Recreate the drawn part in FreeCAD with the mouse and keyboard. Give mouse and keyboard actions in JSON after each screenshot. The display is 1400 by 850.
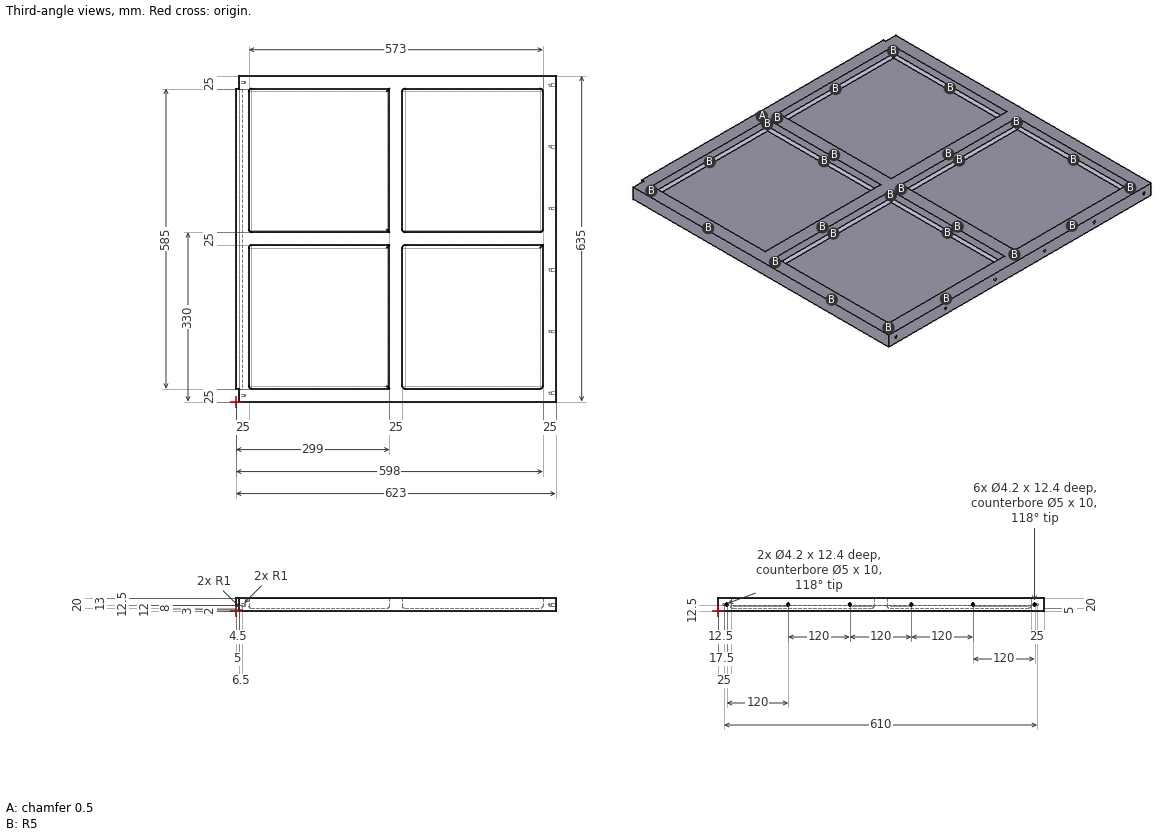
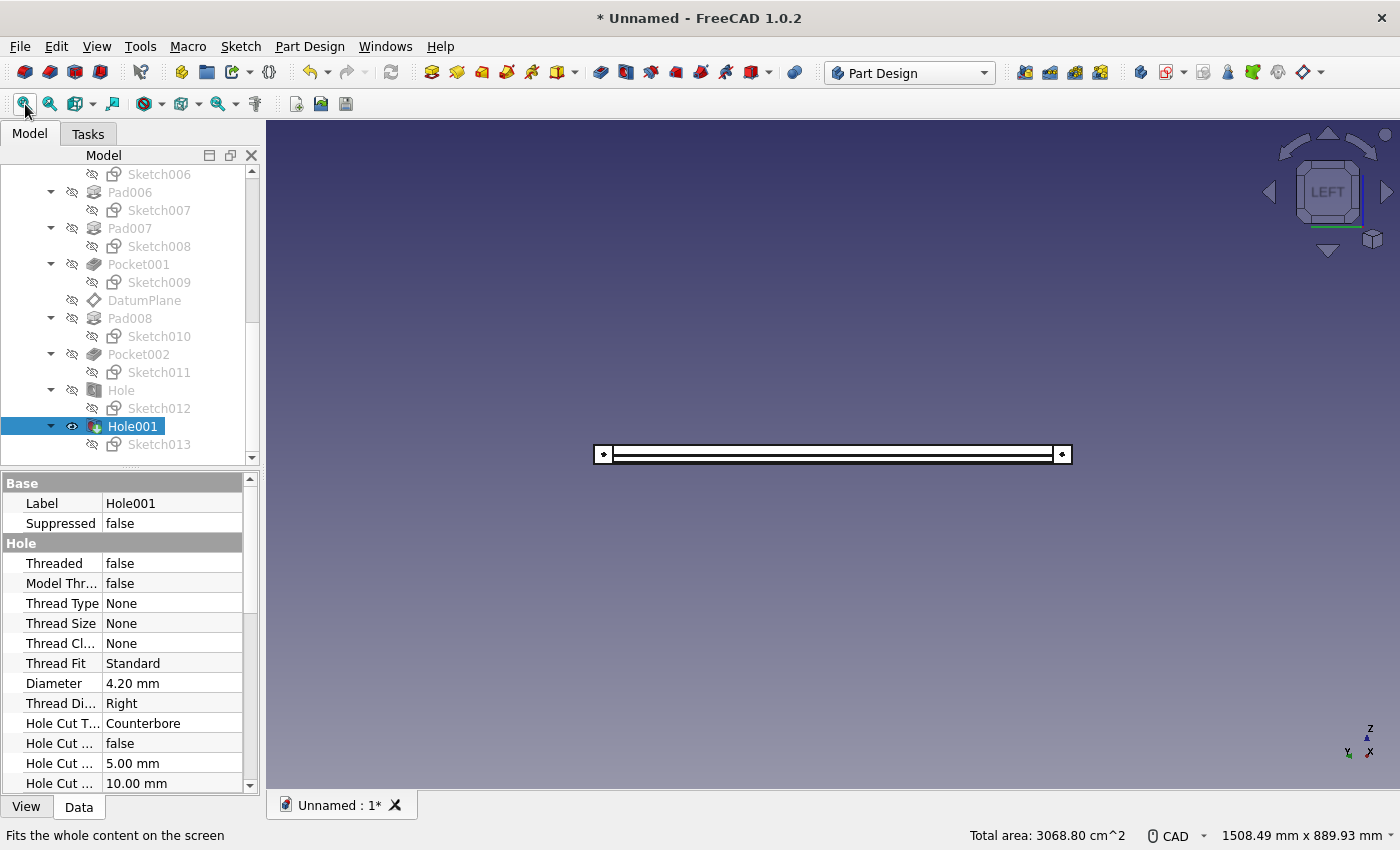
{"action": "scroll", "coordinate": [1053, 452], "scroll_direction": "up", "scroll_amount": 5}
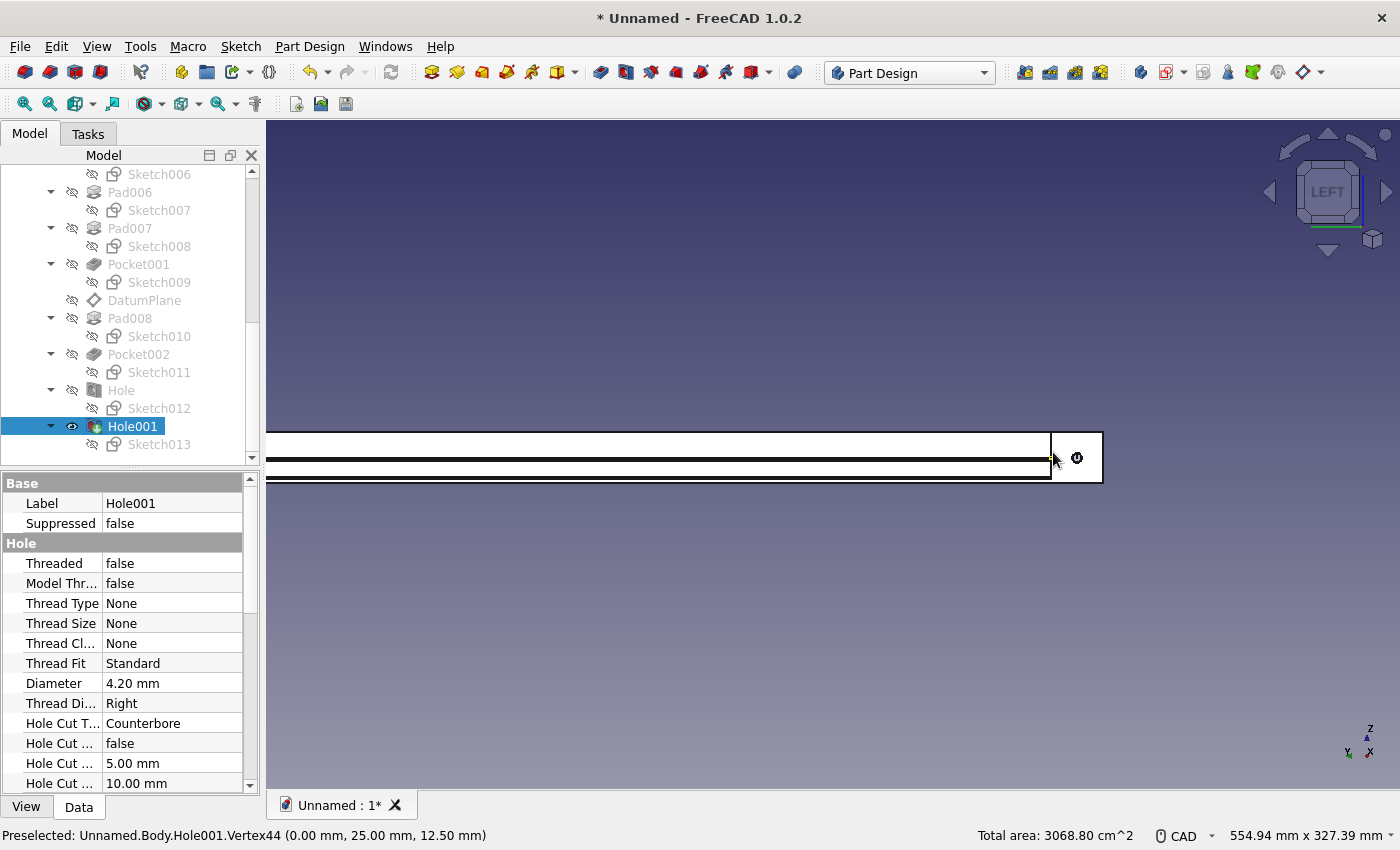
{"action": "left_click", "coordinate": [25, 104]}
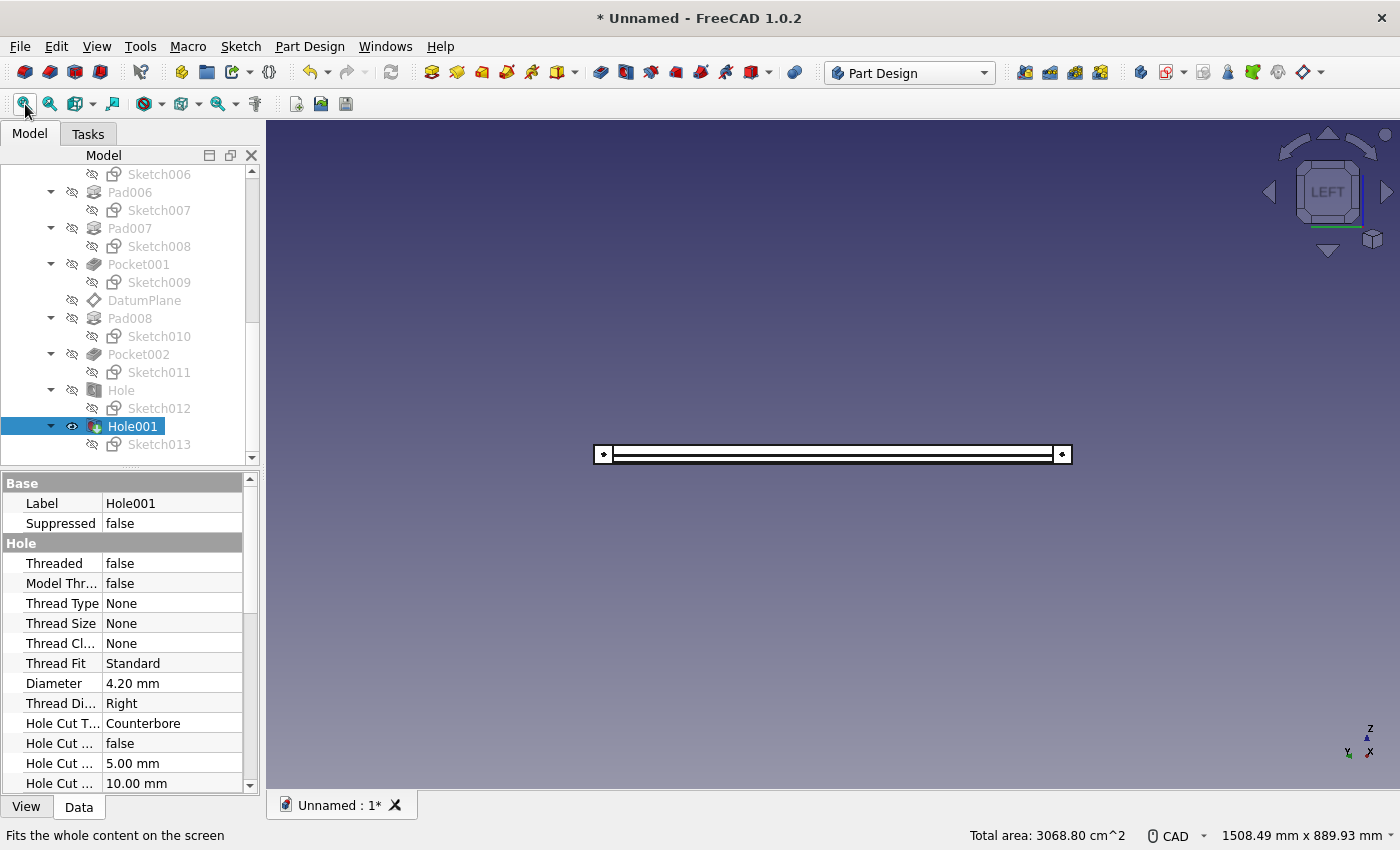
{"action": "key", "text": "v 3"}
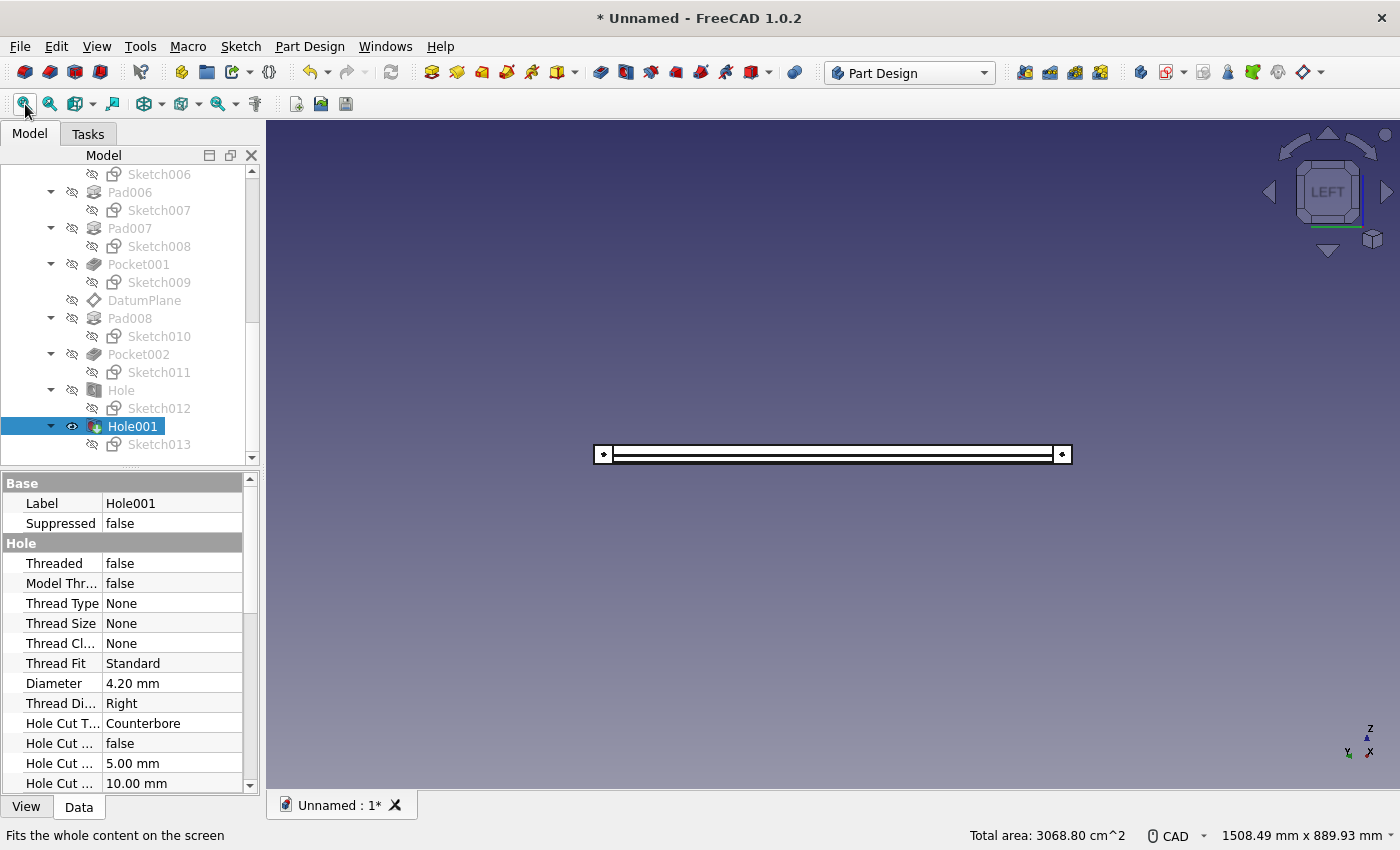
{"action": "key", "text": "0"}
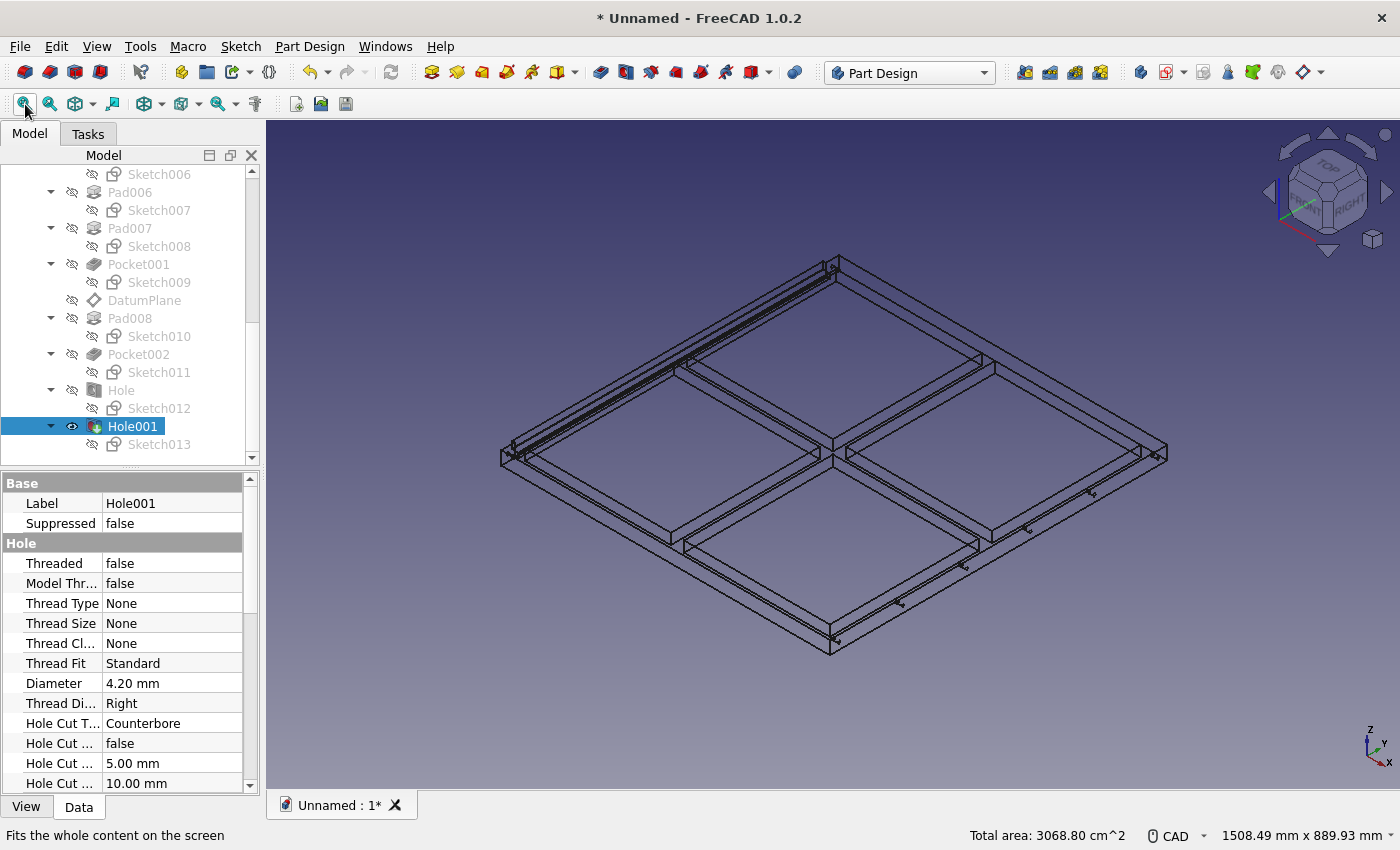
{"action": "left_click", "coordinate": [830, 630], "text": "ctrl"}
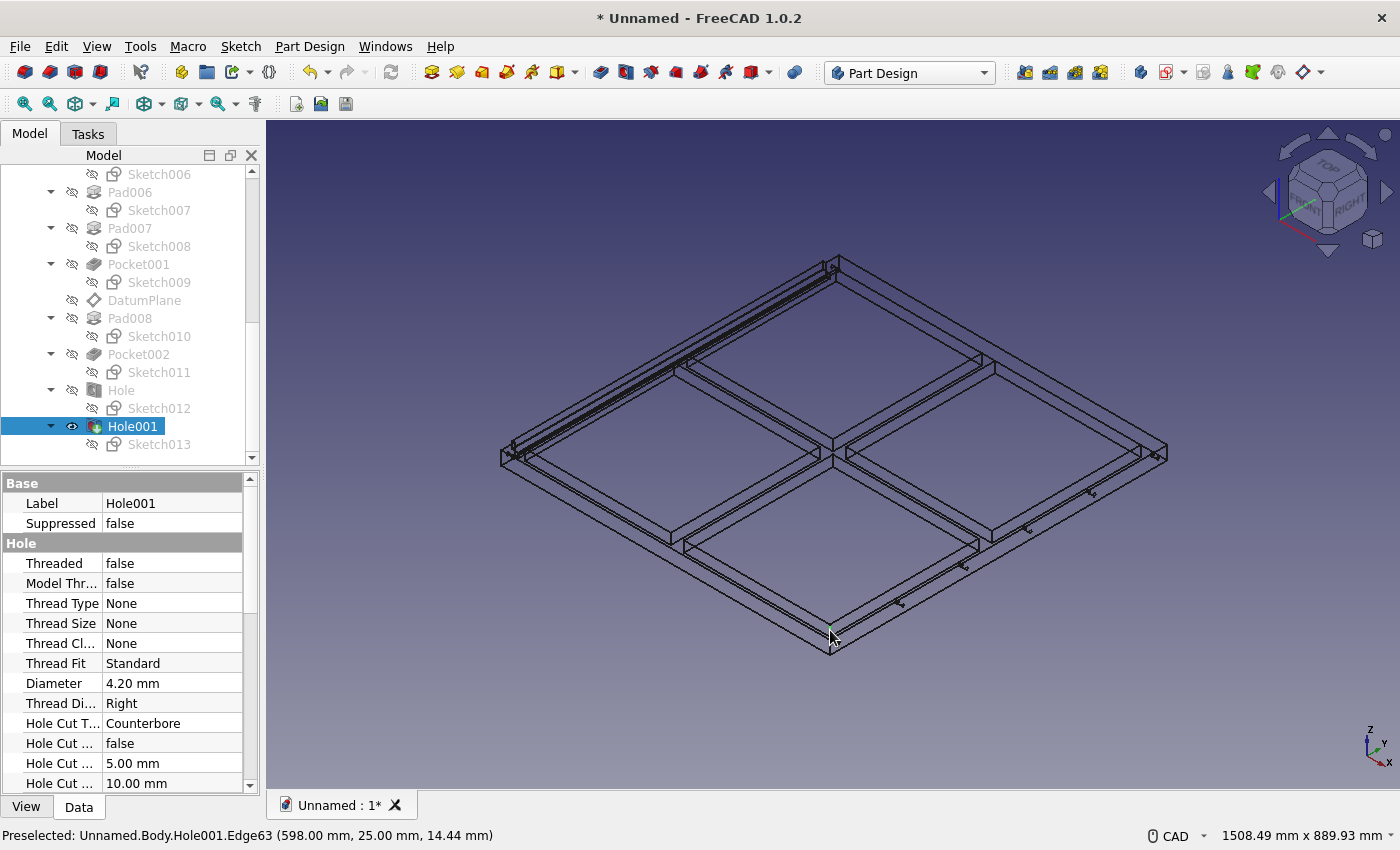
{"action": "left_click", "coordinate": [674, 370], "text": "ctrl"}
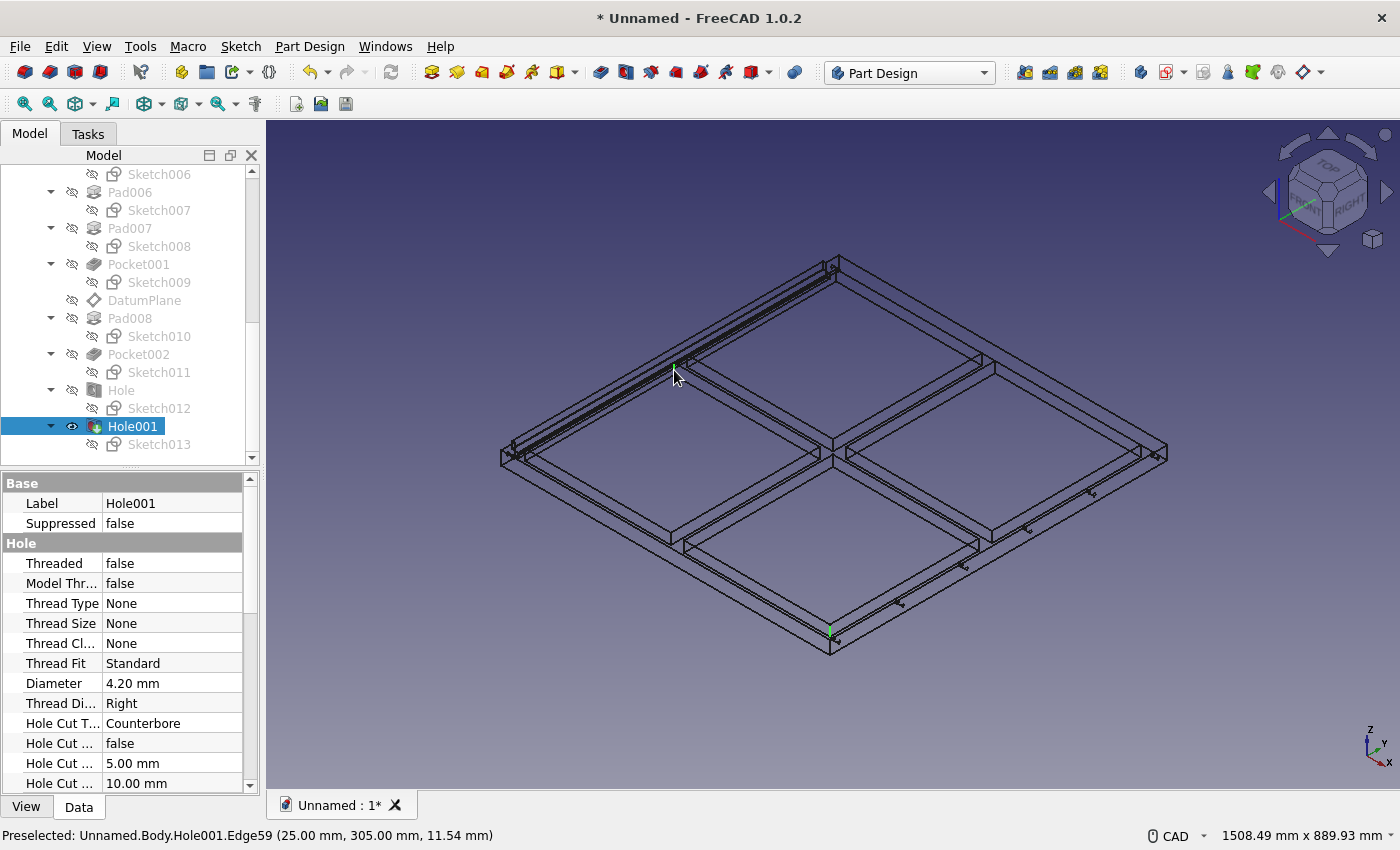
{"action": "left_click", "coordinate": [992, 536], "text": "ctrl"}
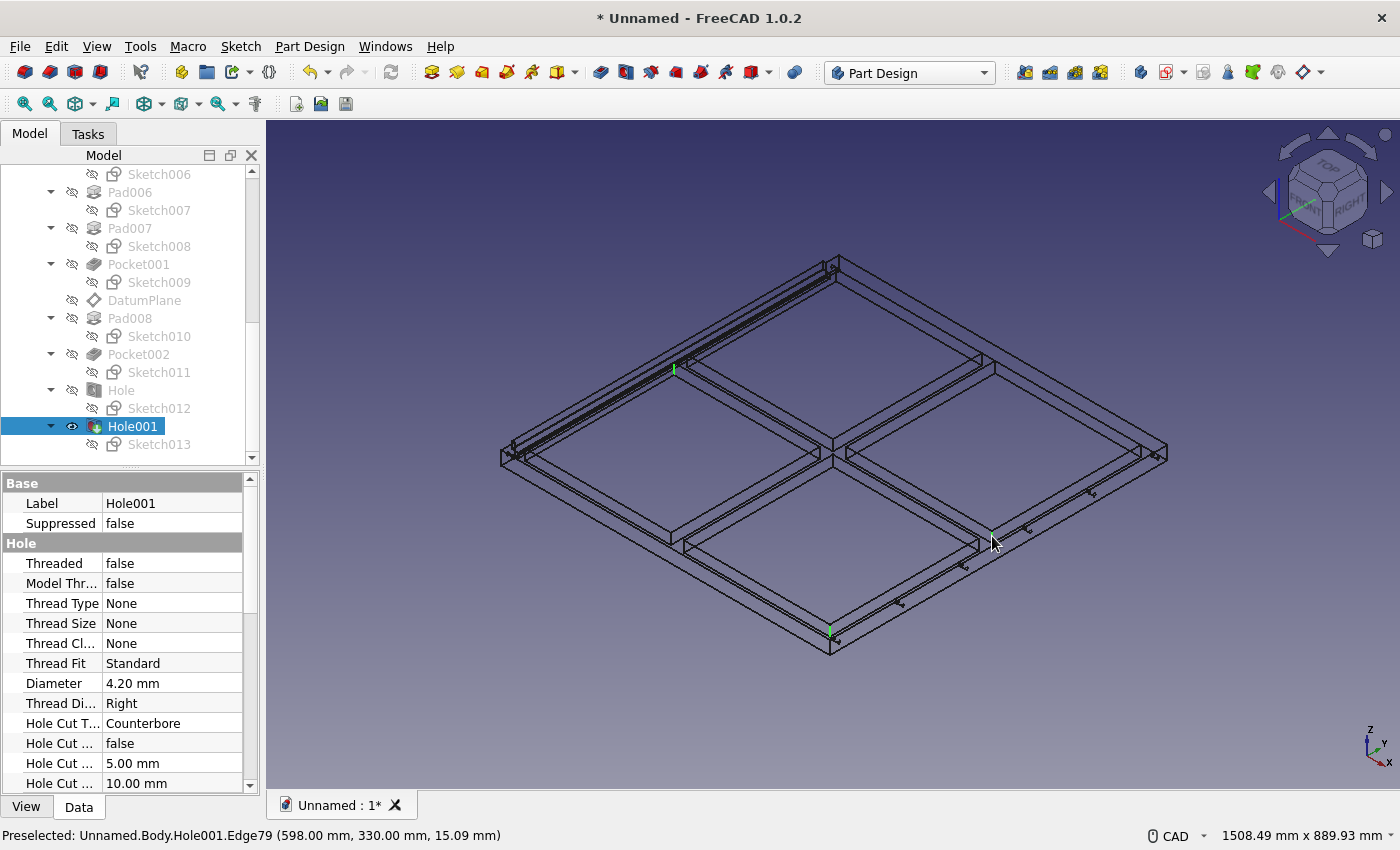
{"action": "left_click", "coordinate": [833, 461], "text": "ctrl"}